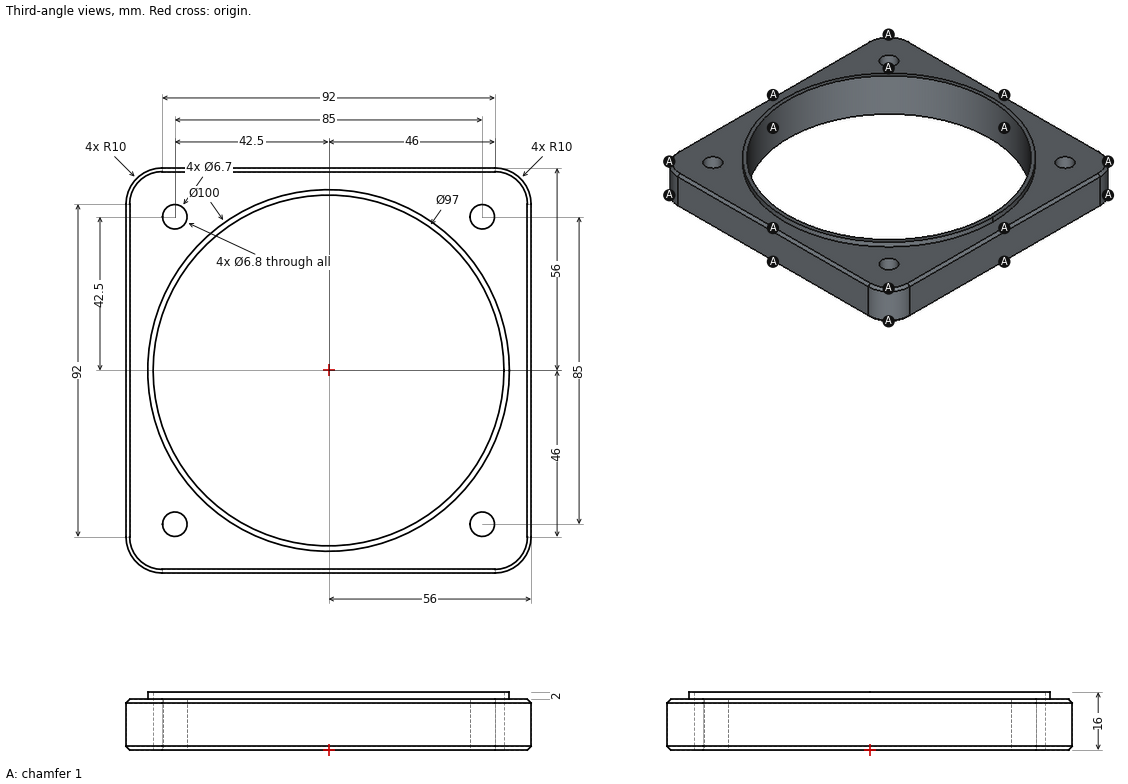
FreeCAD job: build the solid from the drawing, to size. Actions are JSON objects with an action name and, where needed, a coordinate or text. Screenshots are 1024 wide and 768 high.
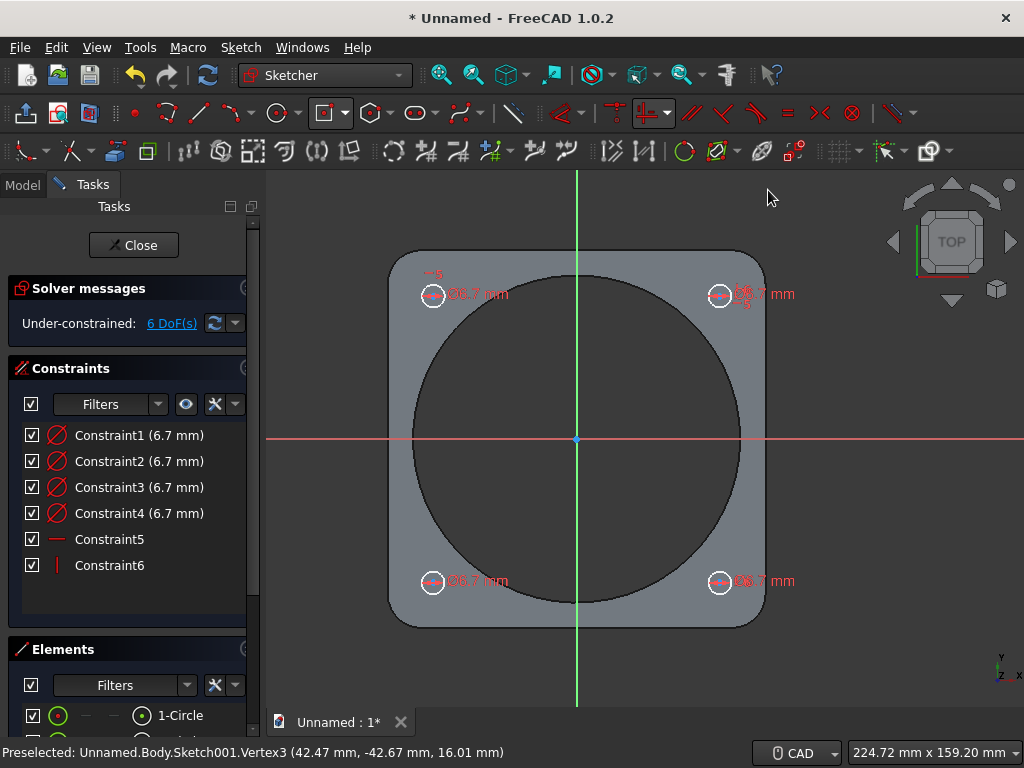
{"action": "left_click", "coordinate": [433, 296]}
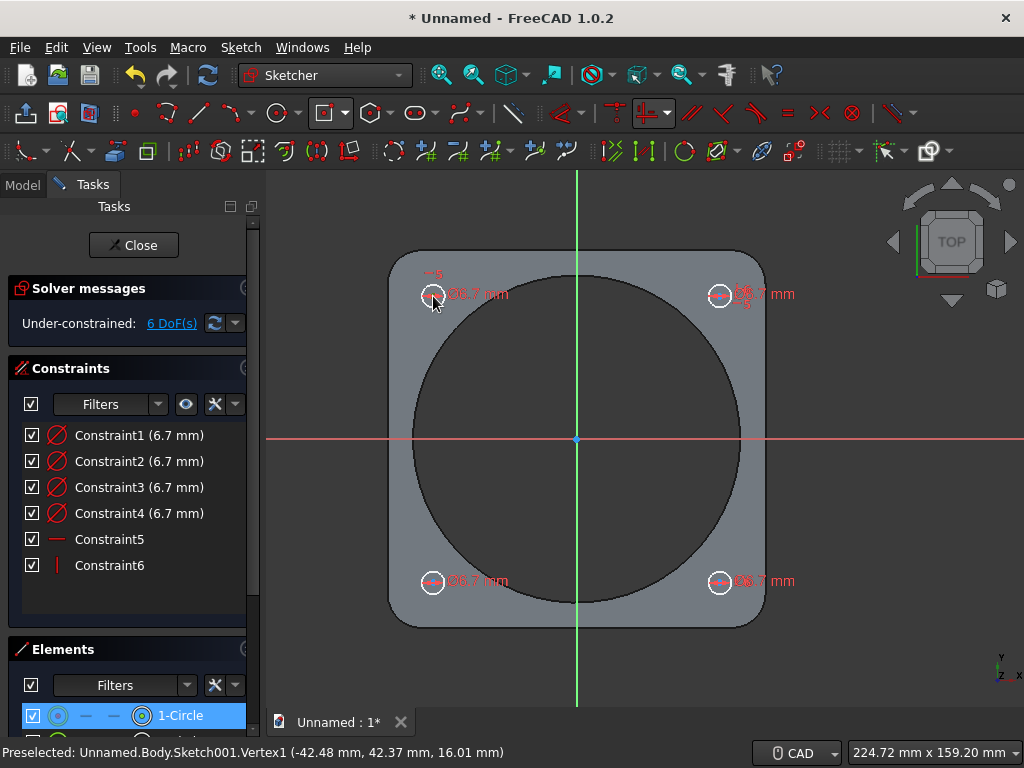
{"action": "left_click", "coordinate": [433, 583]}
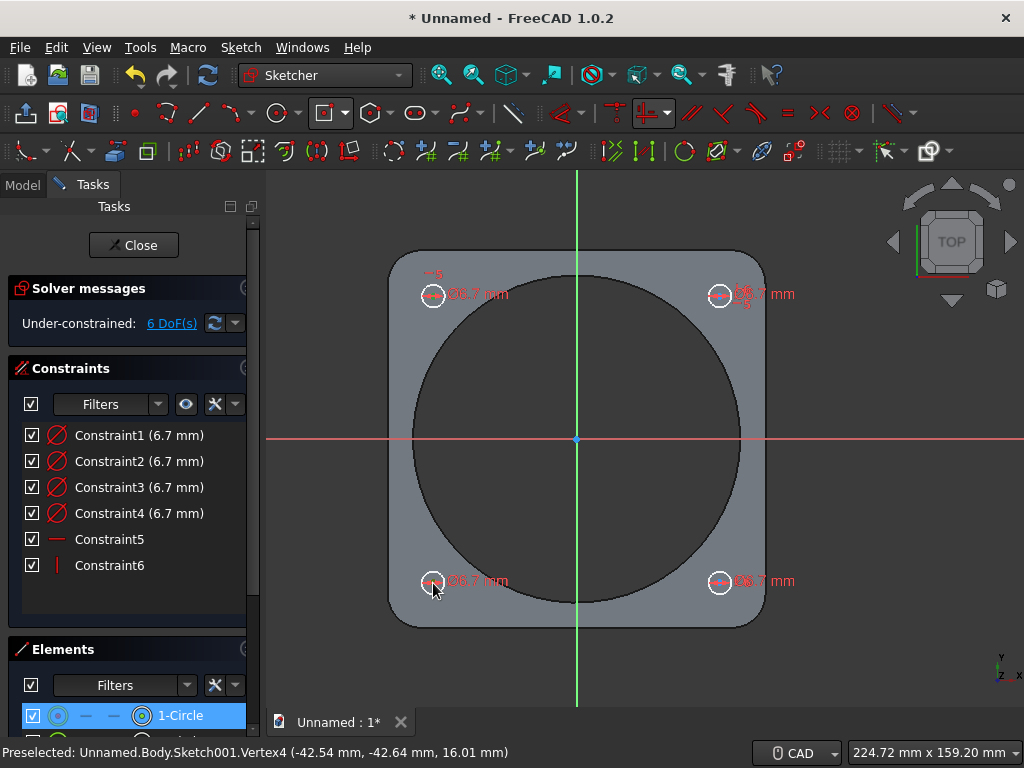
{"action": "key", "text": "v"}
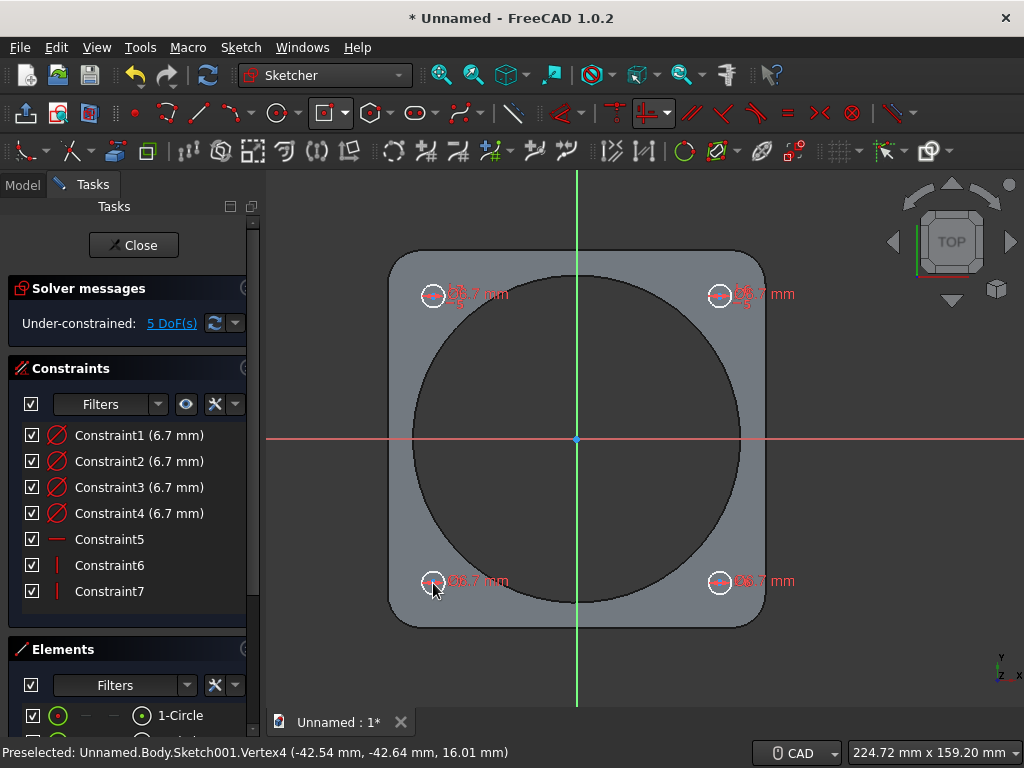
{"action": "left_click", "coordinate": [720, 583]}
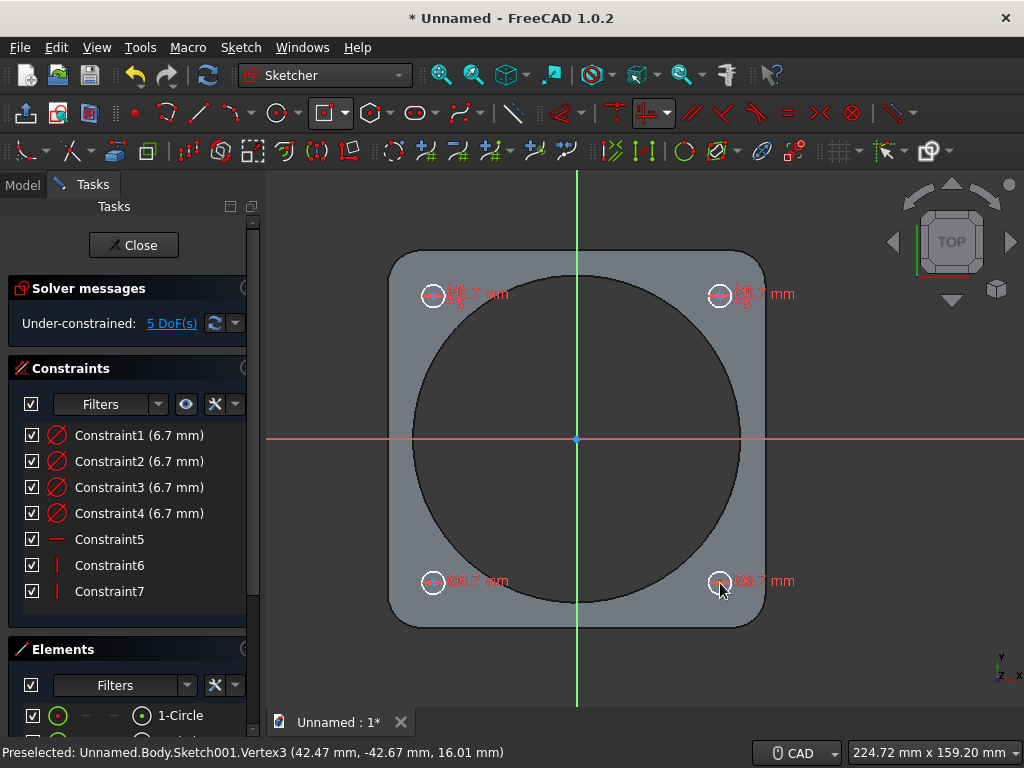
{"action": "left_click", "coordinate": [433, 583]}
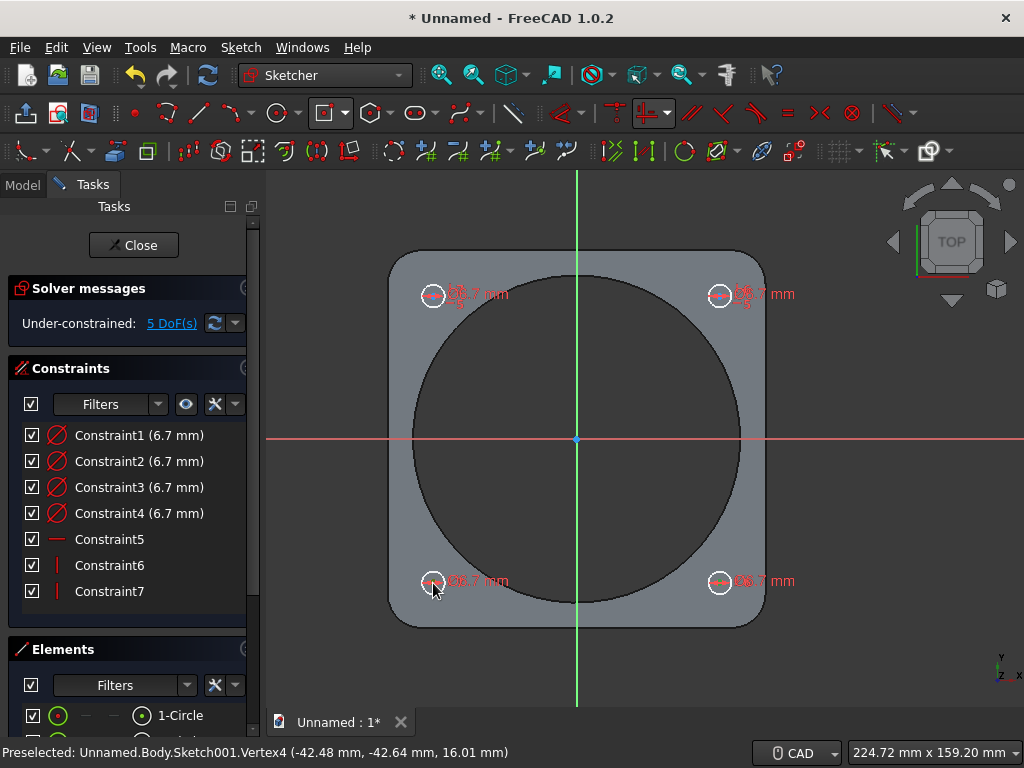
{"action": "key", "text": "h"}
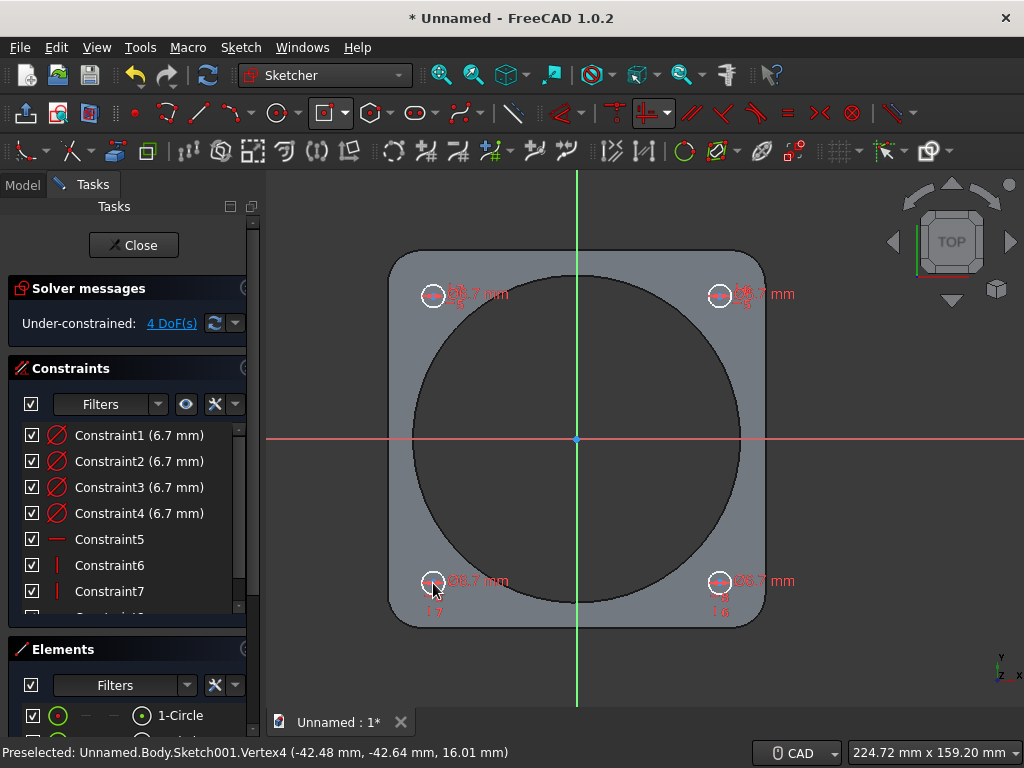
{"action": "left_click", "coordinate": [560, 114]}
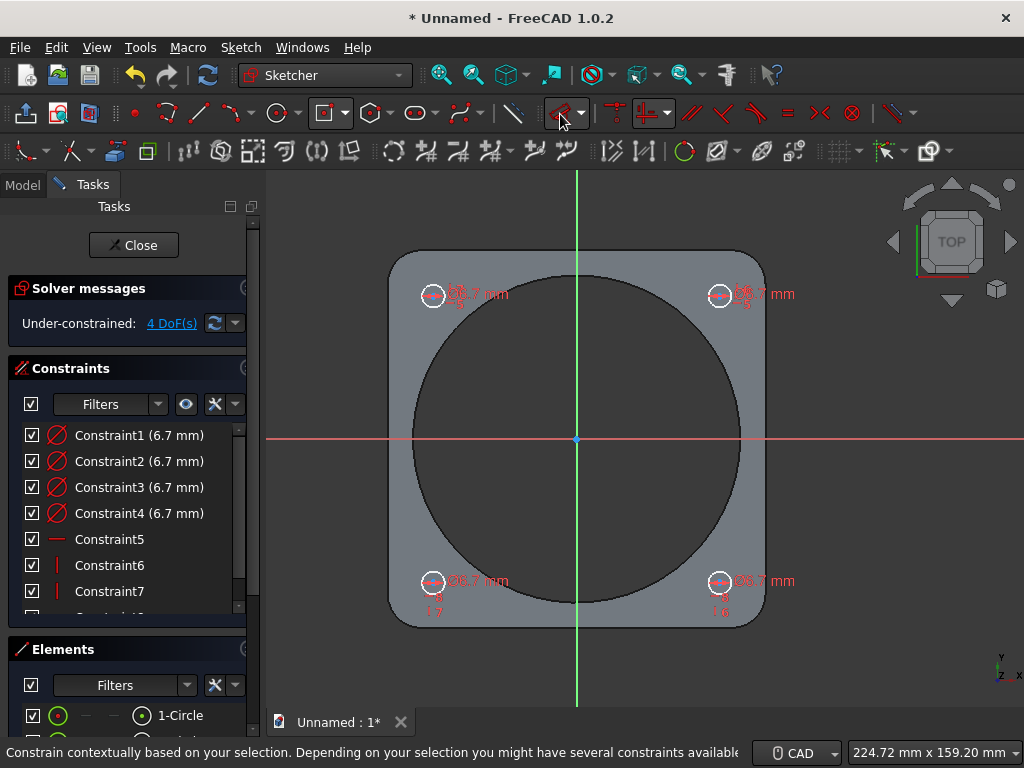
{"action": "left_click", "coordinate": [433, 296]}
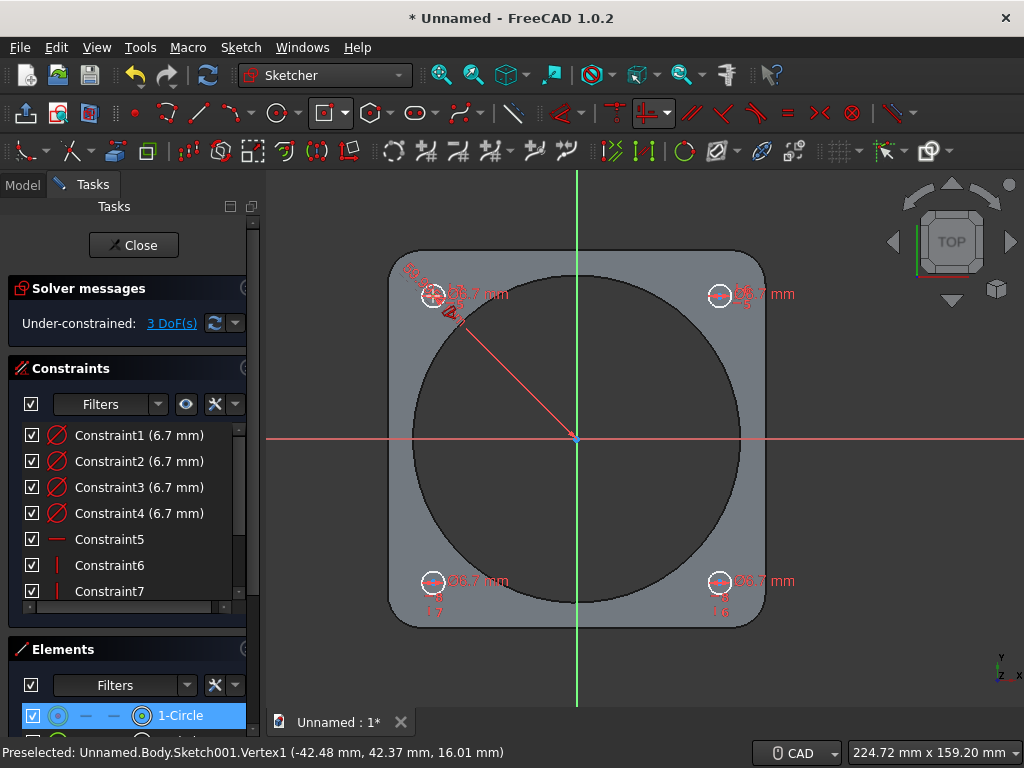
{"action": "left_click", "coordinate": [720, 296]}
{"action": "left_click", "coordinate": [511, 262]}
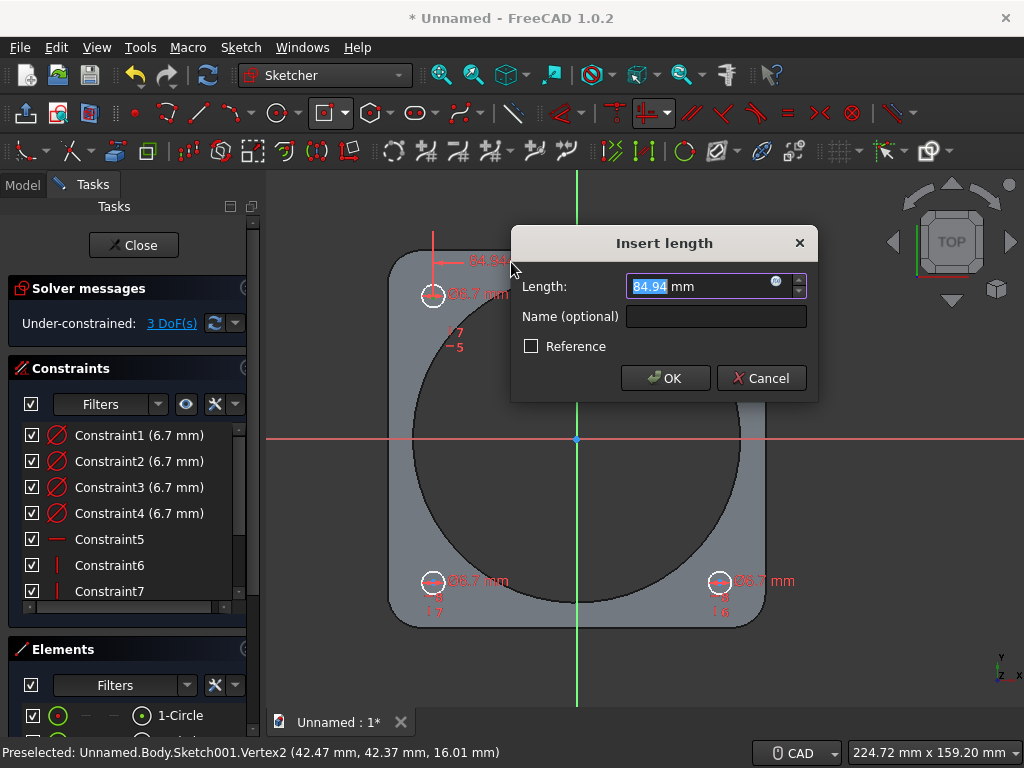
{"action": "type", "text": "85"}
{"action": "key", "text": "Return"}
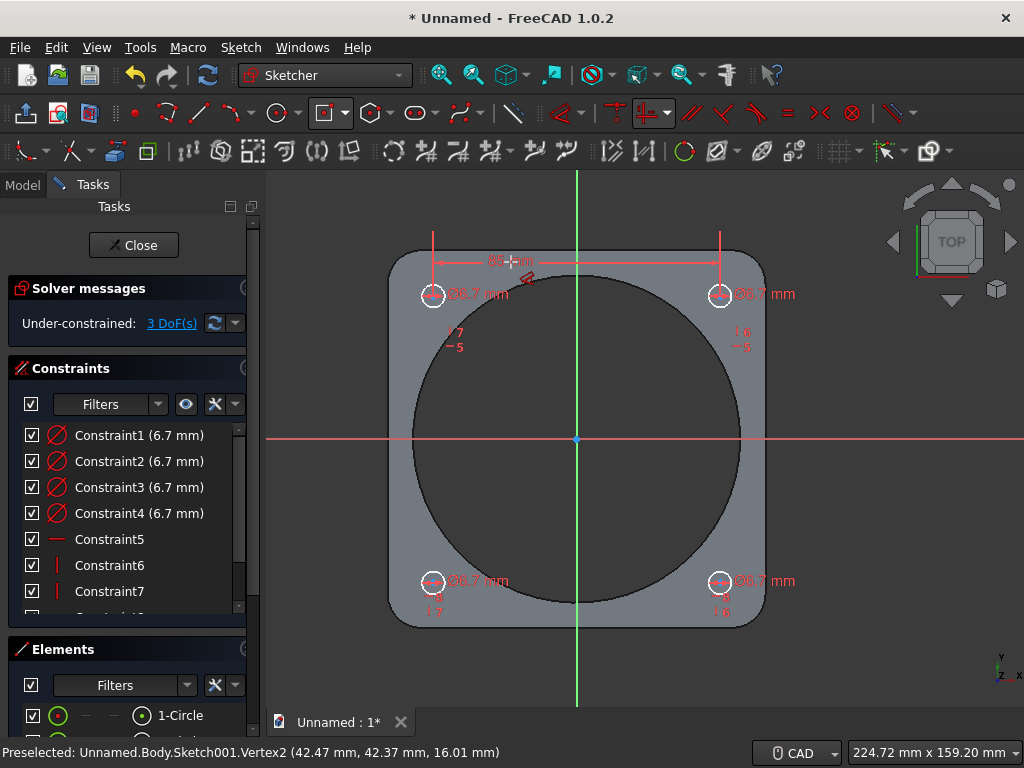
{"action": "left_click", "coordinate": [720, 296]}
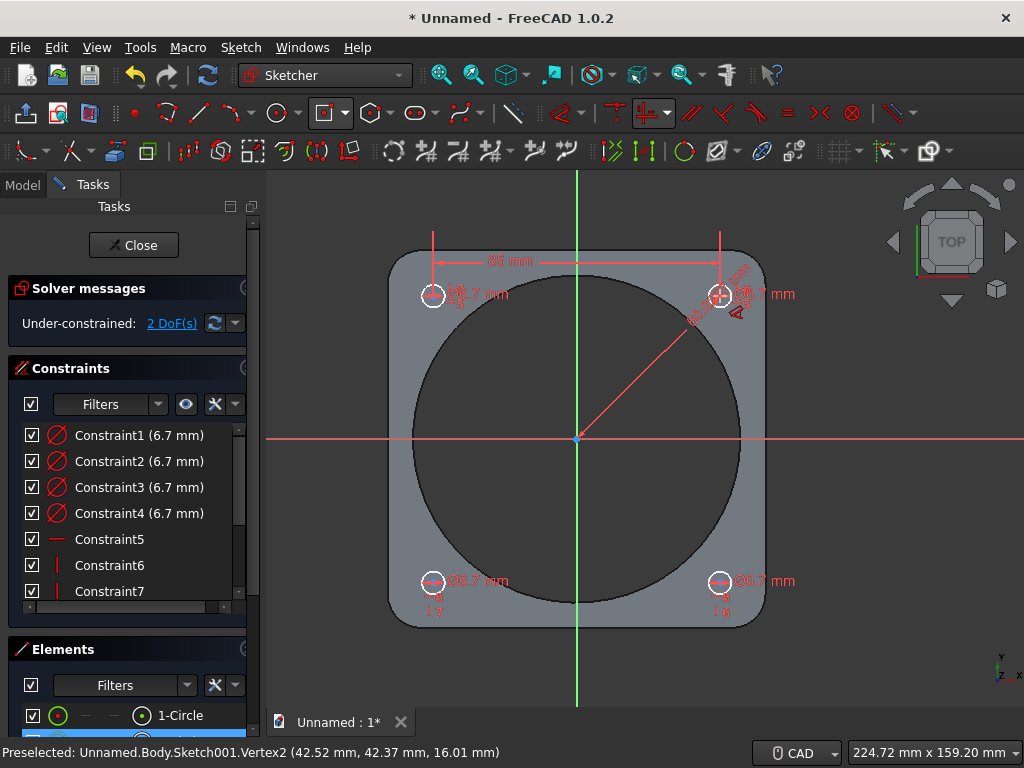
{"action": "left_click", "coordinate": [720, 583]}
{"action": "left_click", "coordinate": [754, 374]}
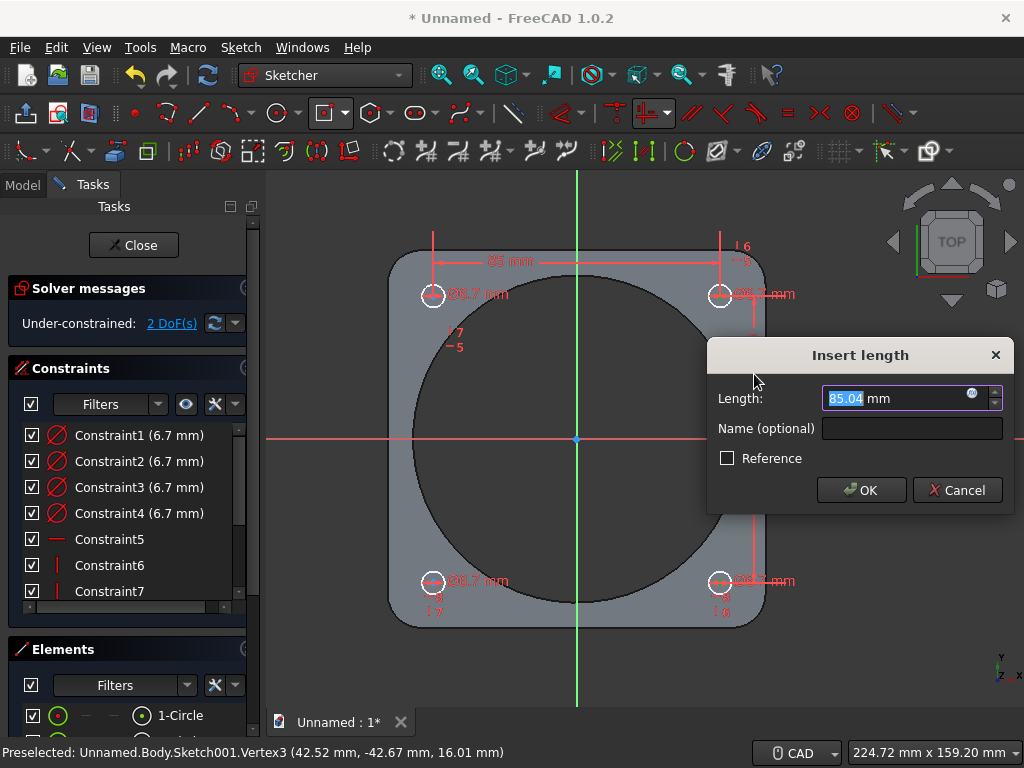
{"action": "type", "text": "85"}
{"action": "key", "text": "Return"}